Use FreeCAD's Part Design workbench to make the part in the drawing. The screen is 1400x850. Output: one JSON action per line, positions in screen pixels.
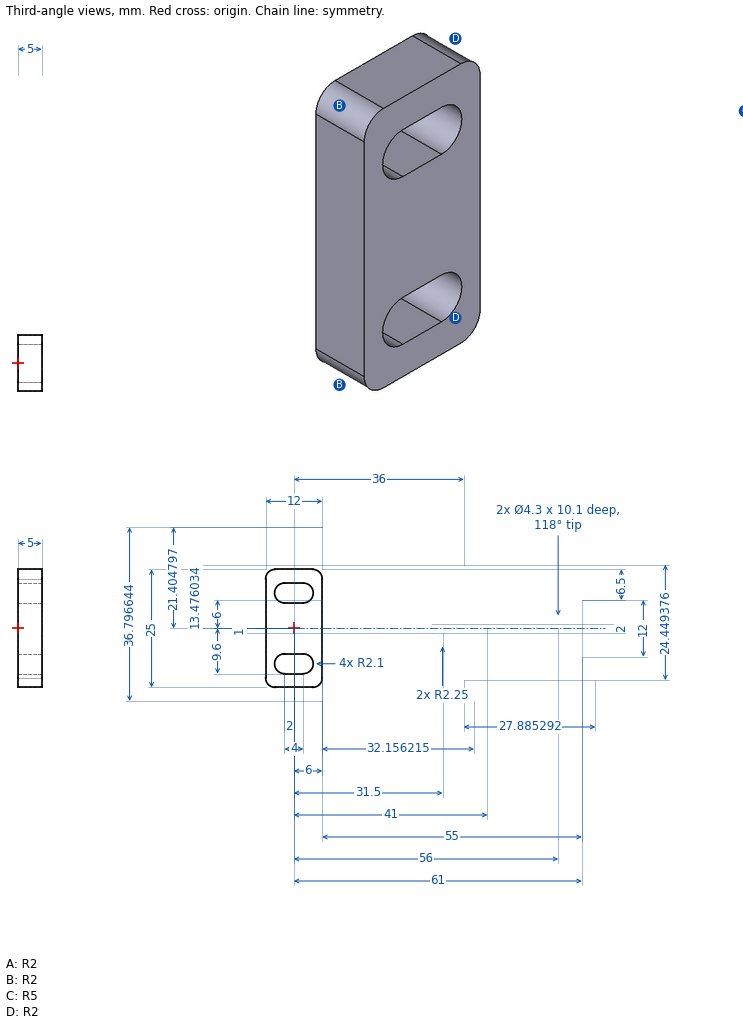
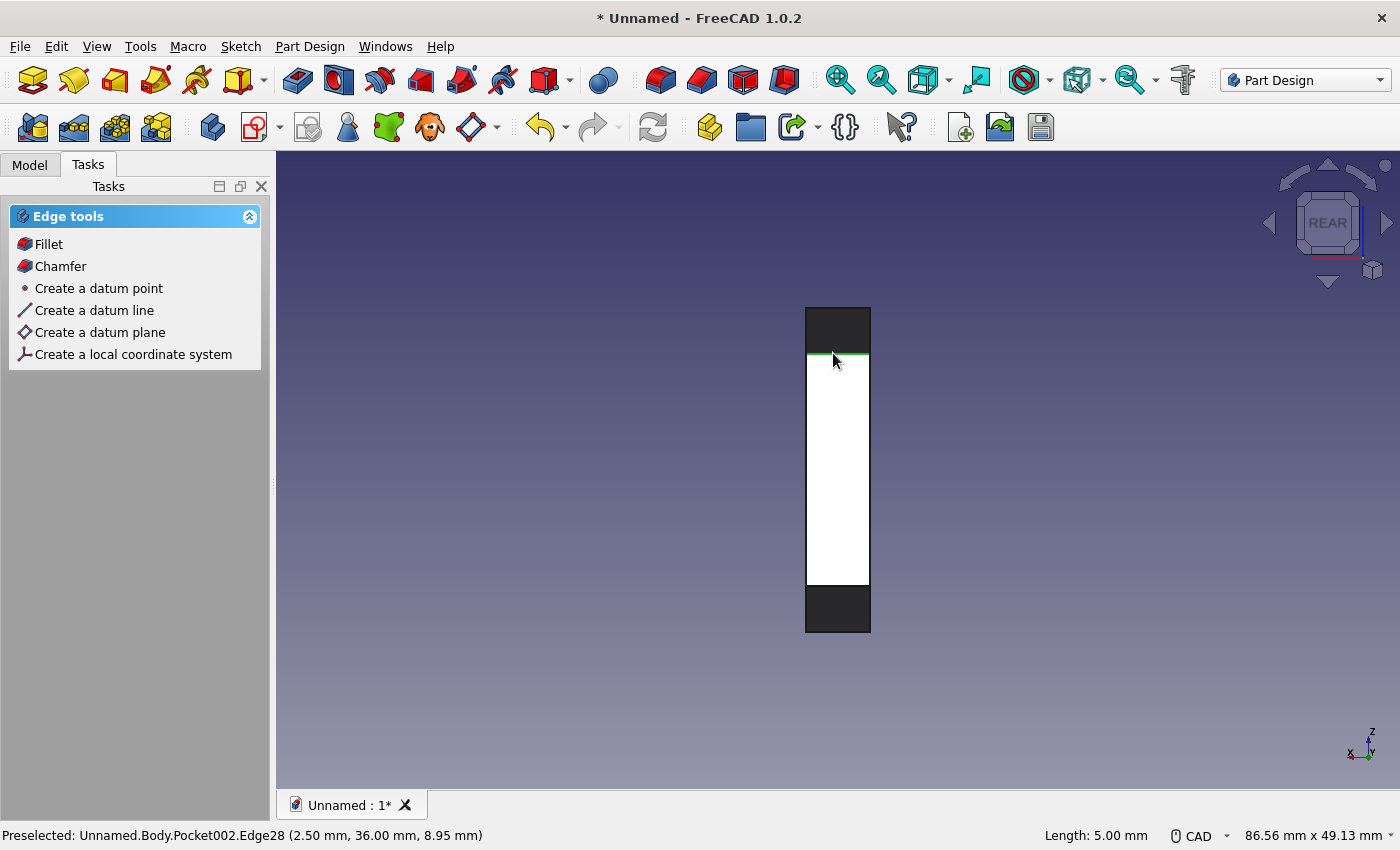
{"action": "left_click", "coordinate": [838, 585], "text": "ctrl"}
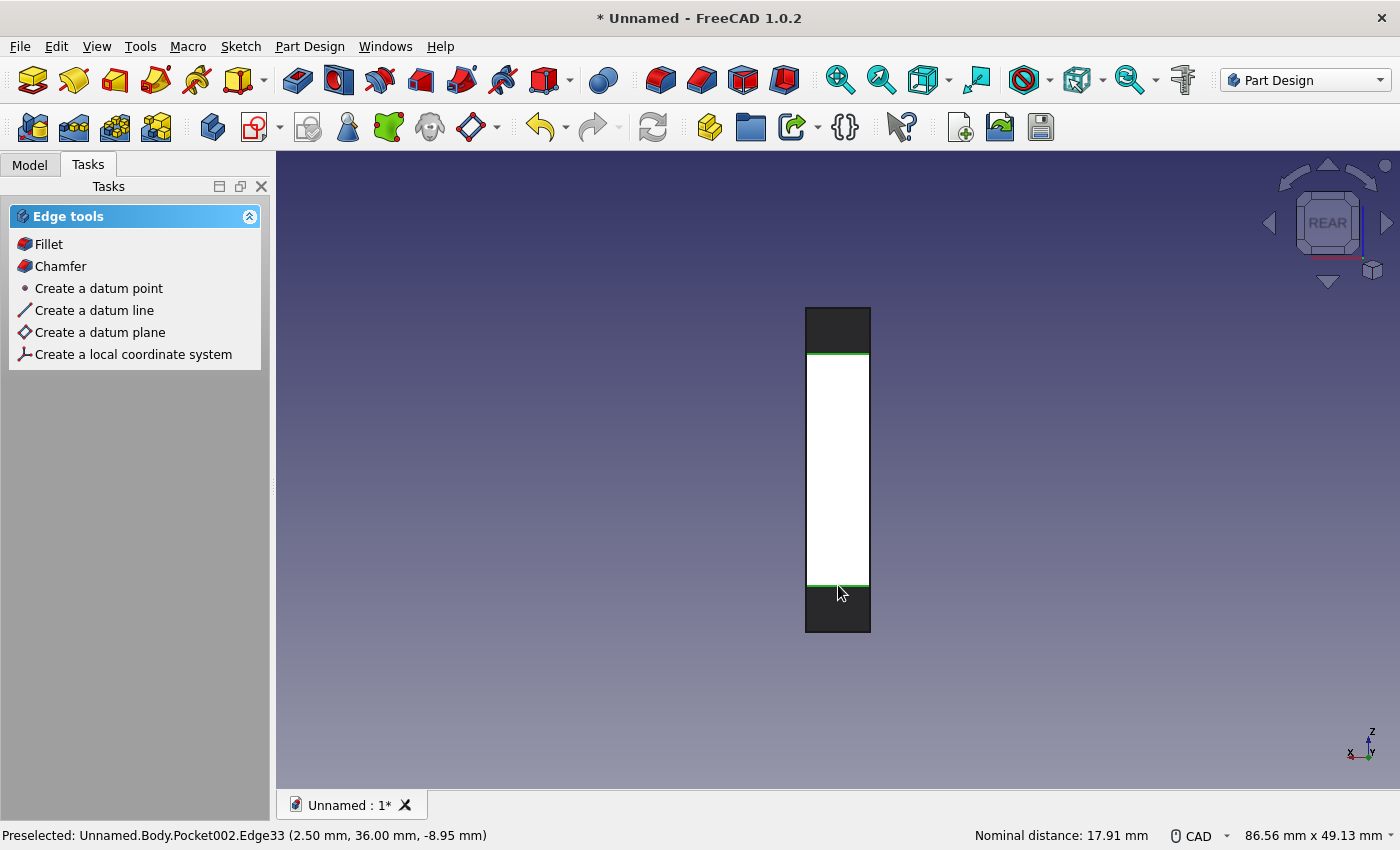
{"action": "left_click", "coordinate": [661, 80]}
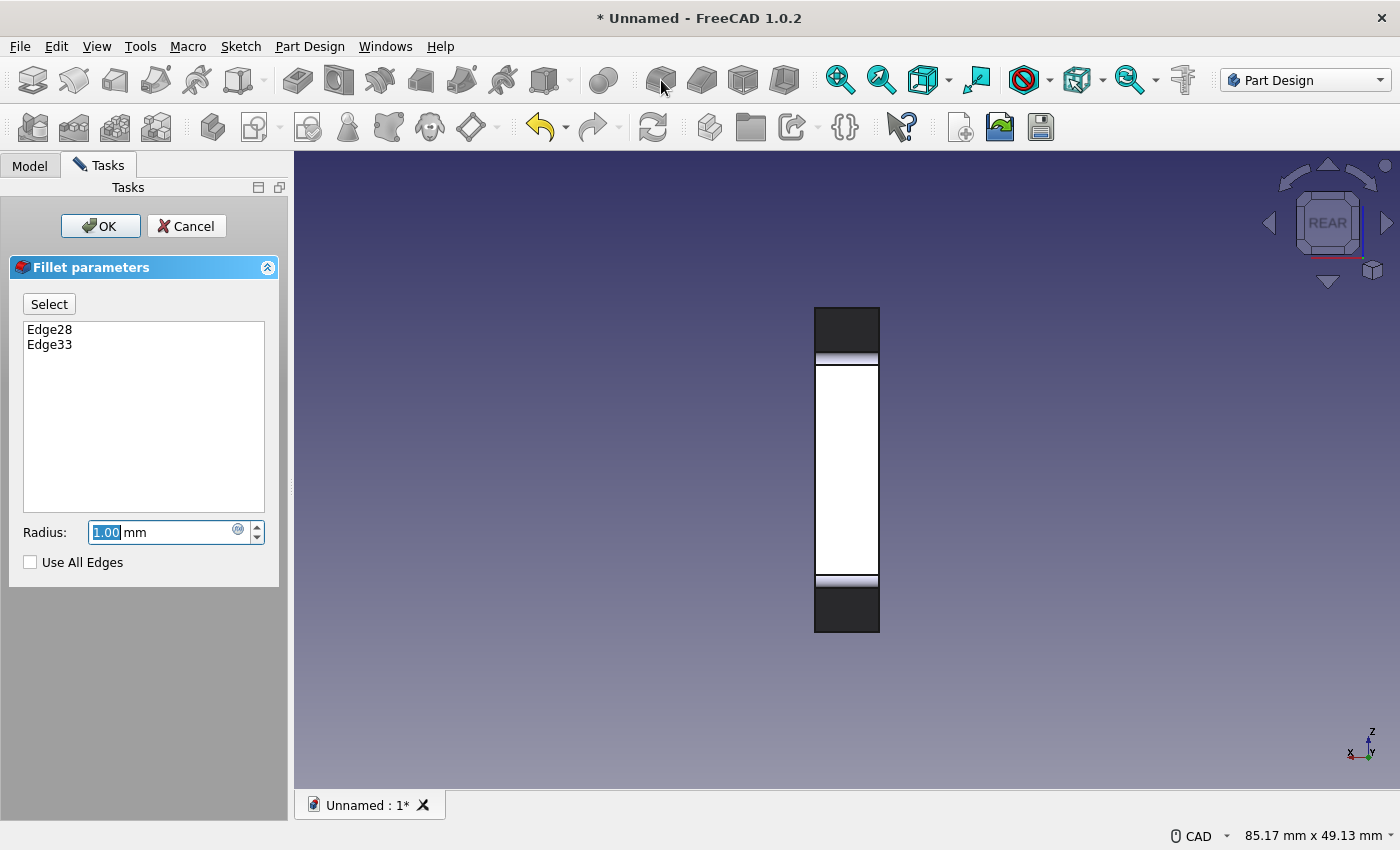
{"action": "type", "text": "5"}
{"action": "key", "text": "Tab"}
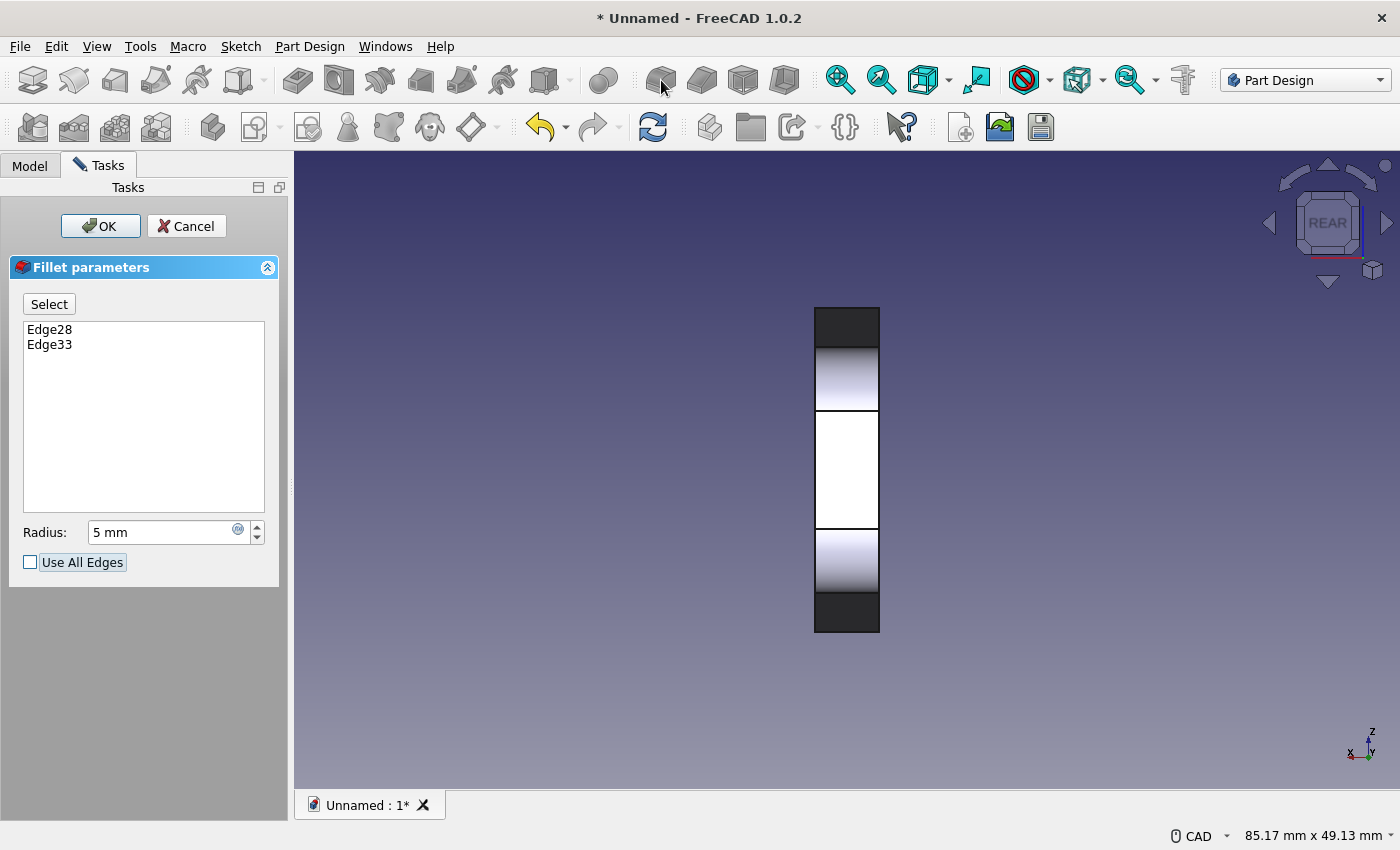
{"action": "left_click", "coordinate": [101, 226]}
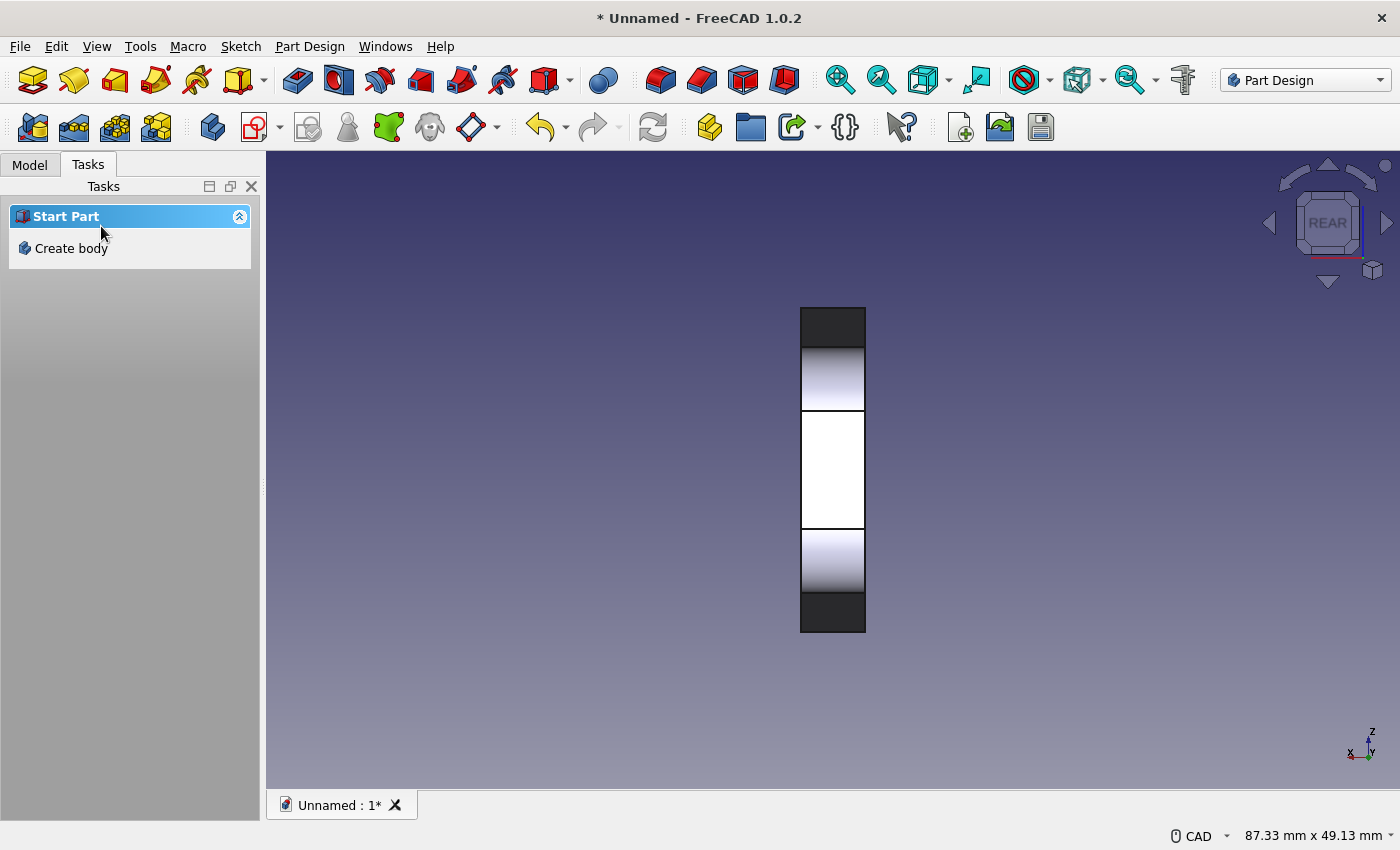
{"action": "key", "text": "0"}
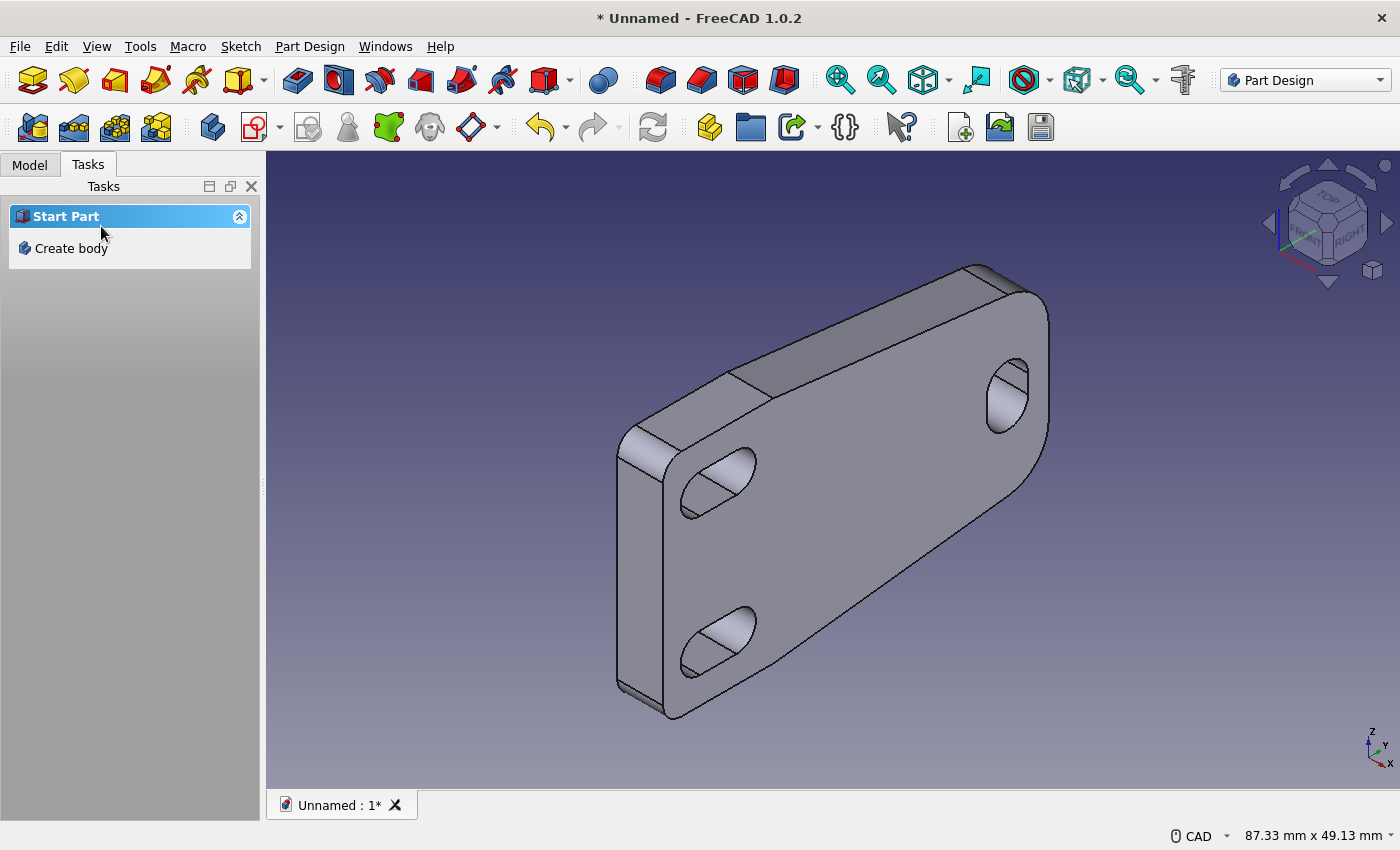
{"action": "left_click", "coordinate": [856, 482]}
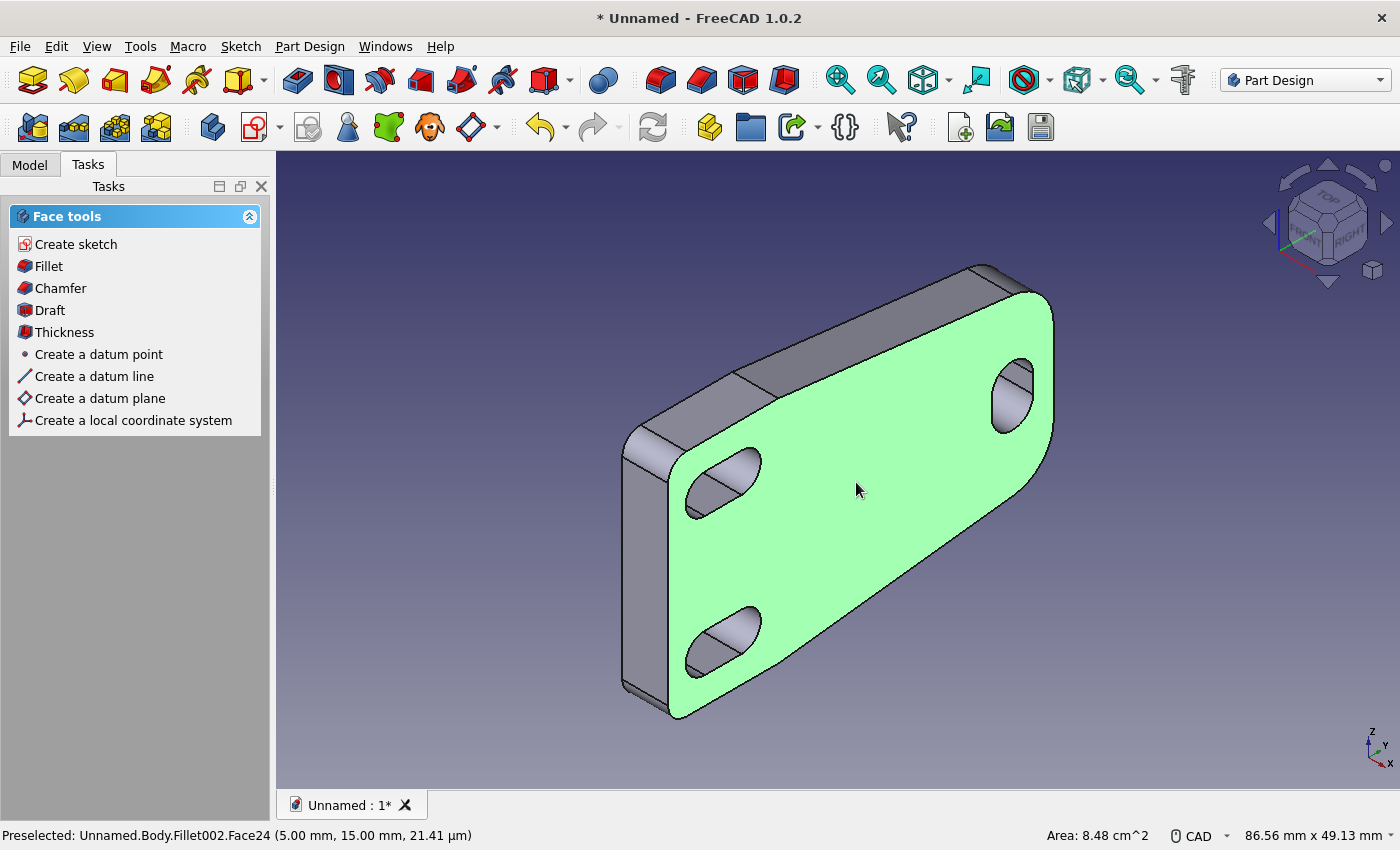
{"action": "left_click", "coordinate": [254, 128]}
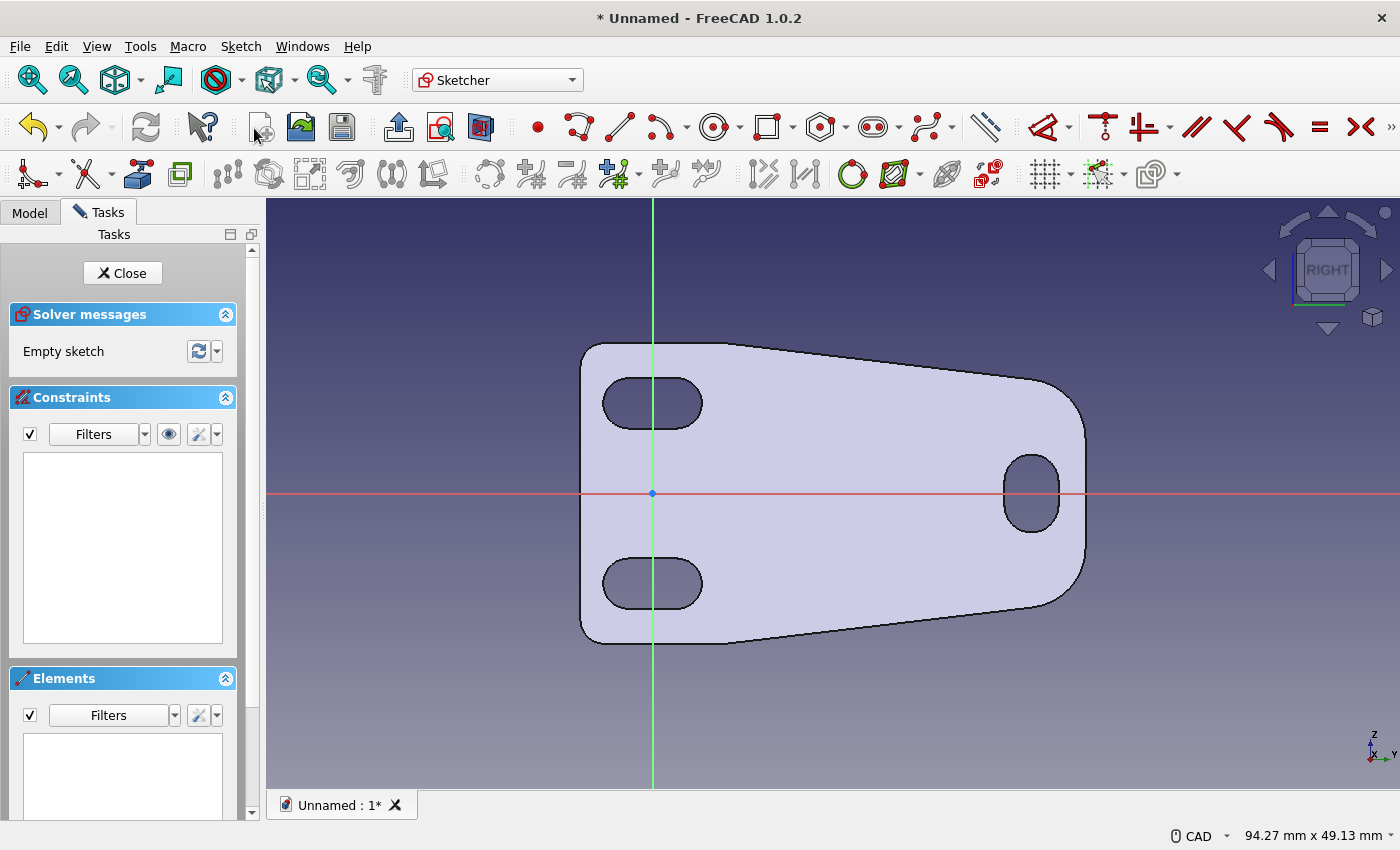
{"action": "scroll", "coordinate": [294, 657], "scroll_direction": "down", "scroll_amount": 1}